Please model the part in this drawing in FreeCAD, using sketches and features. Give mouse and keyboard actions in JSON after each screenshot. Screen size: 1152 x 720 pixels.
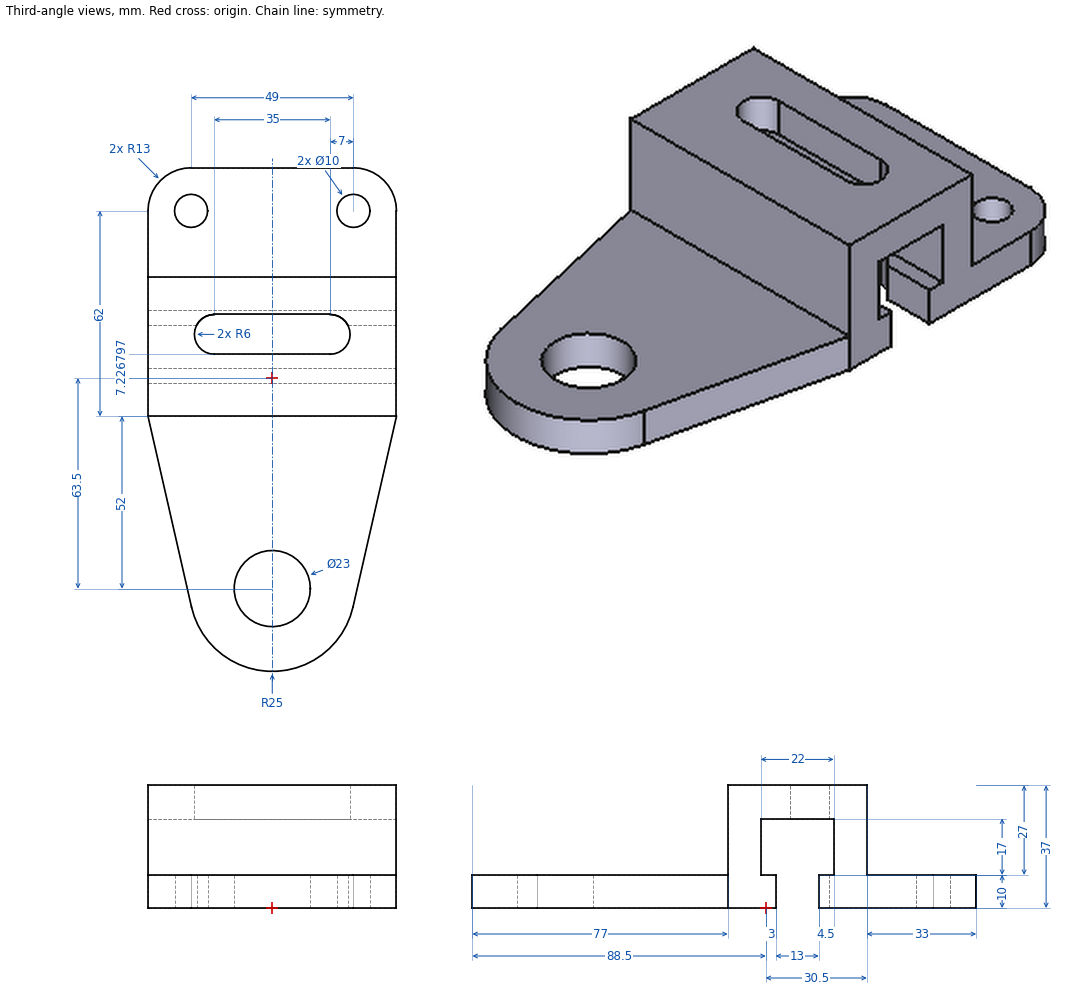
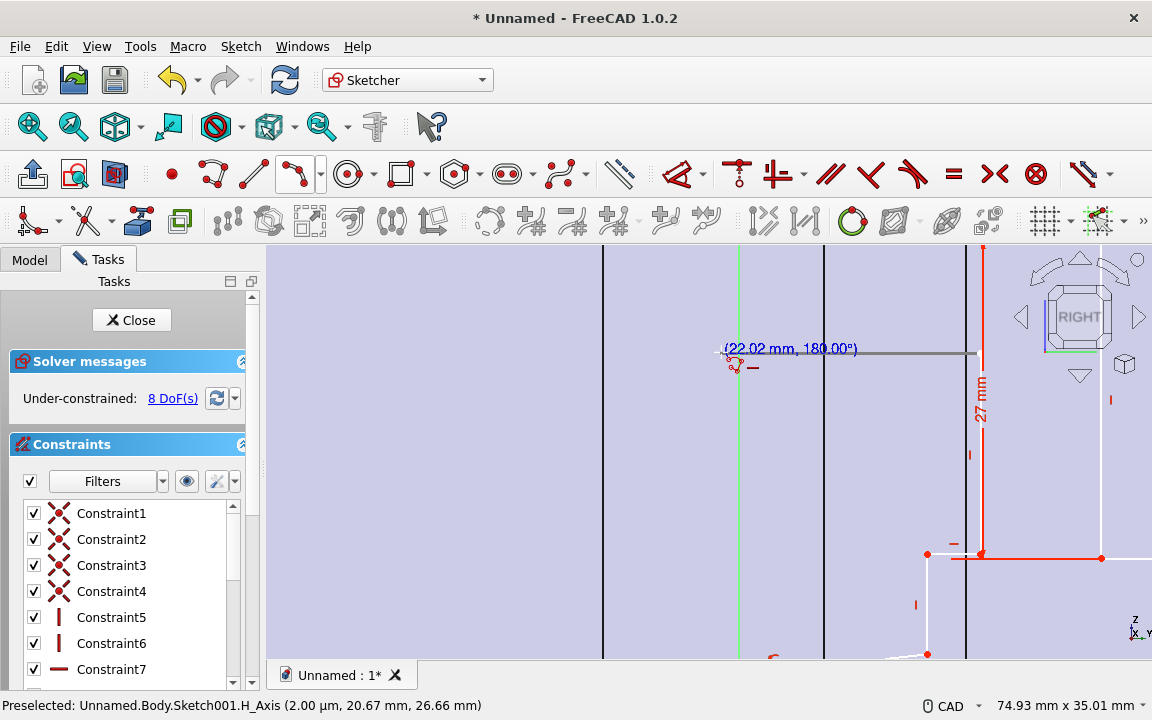
{"action": "left_click", "coordinate": [721, 352]}
{"action": "left_click", "coordinate": [721, 553]}
{"action": "left_click", "coordinate": [774, 553]}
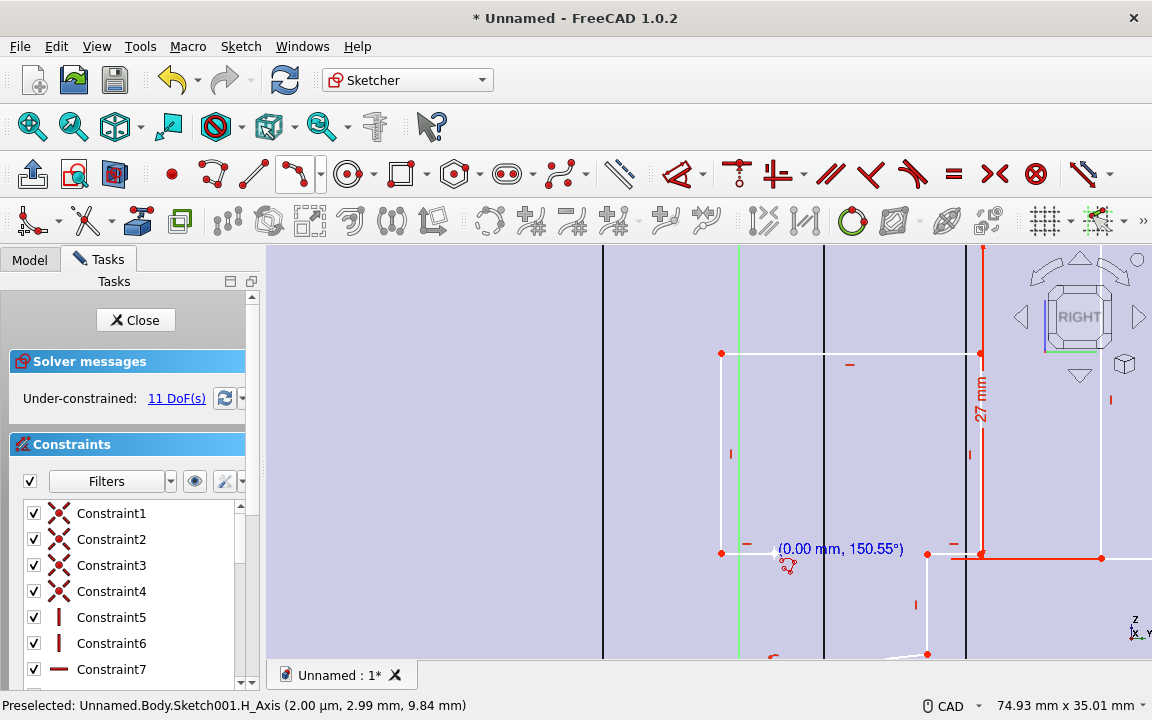
{"action": "scroll", "coordinate": [657, 452], "scroll_direction": "down", "scroll_amount": 7}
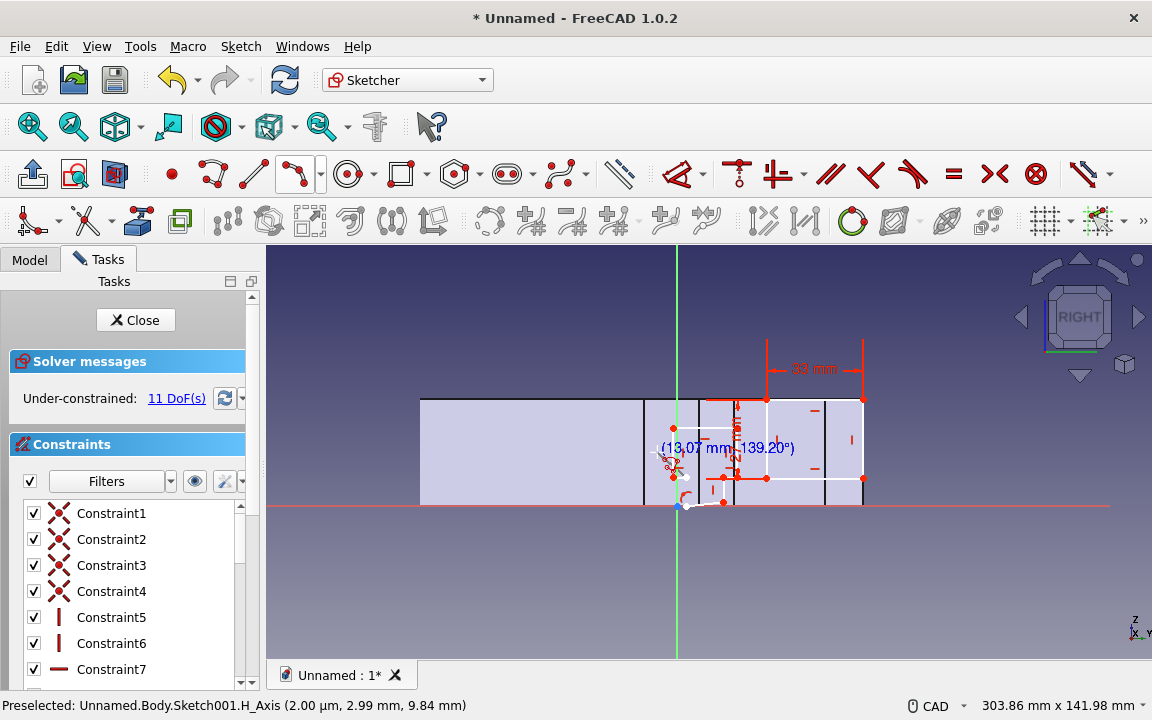
{"action": "scroll", "coordinate": [686, 506], "scroll_direction": "up", "scroll_amount": 3}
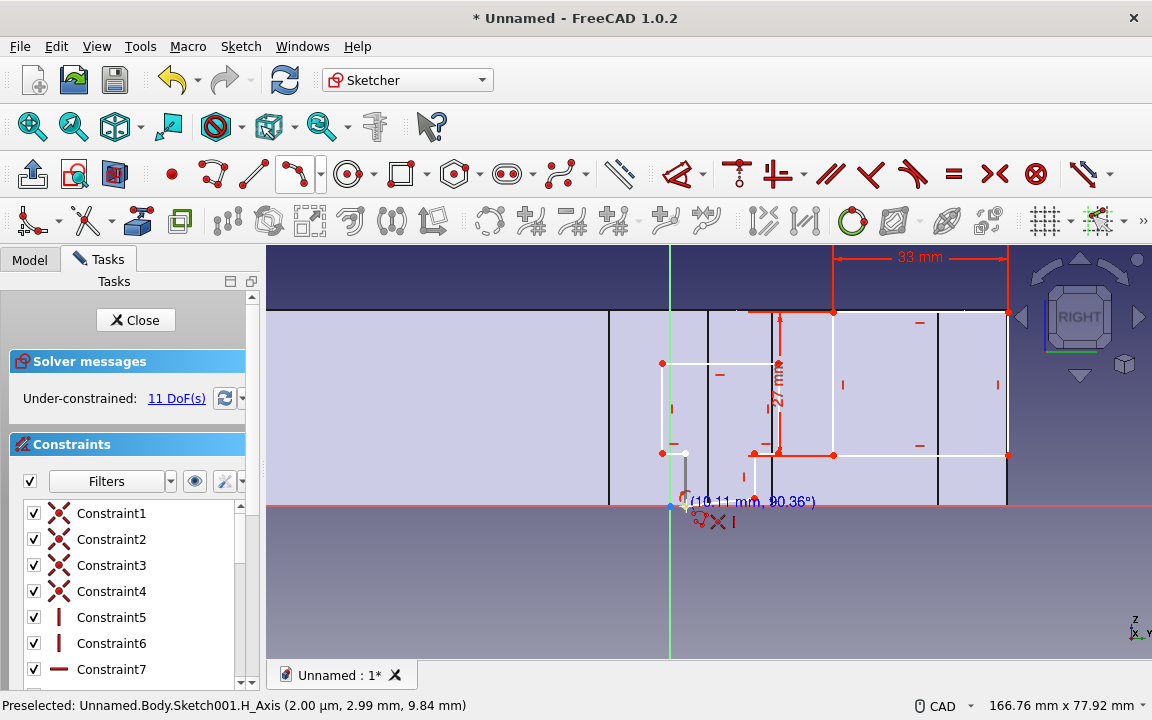
{"action": "left_click", "coordinate": [686, 506]}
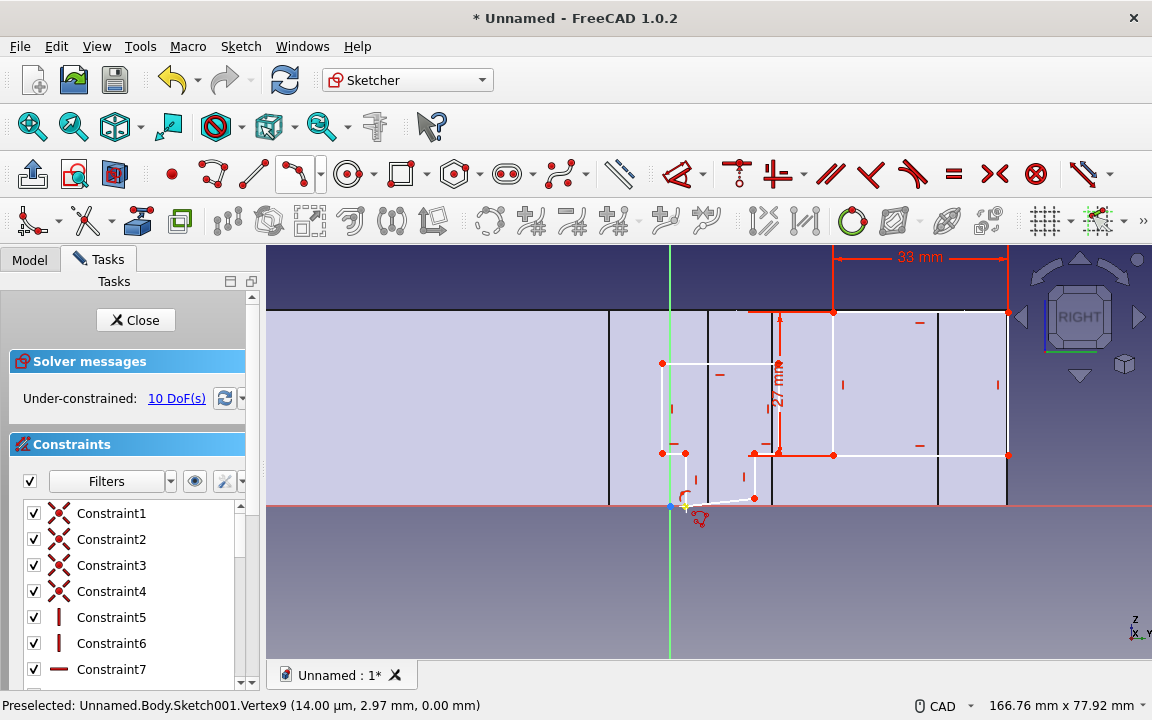
{"action": "left_click", "coordinate": [400, 174]}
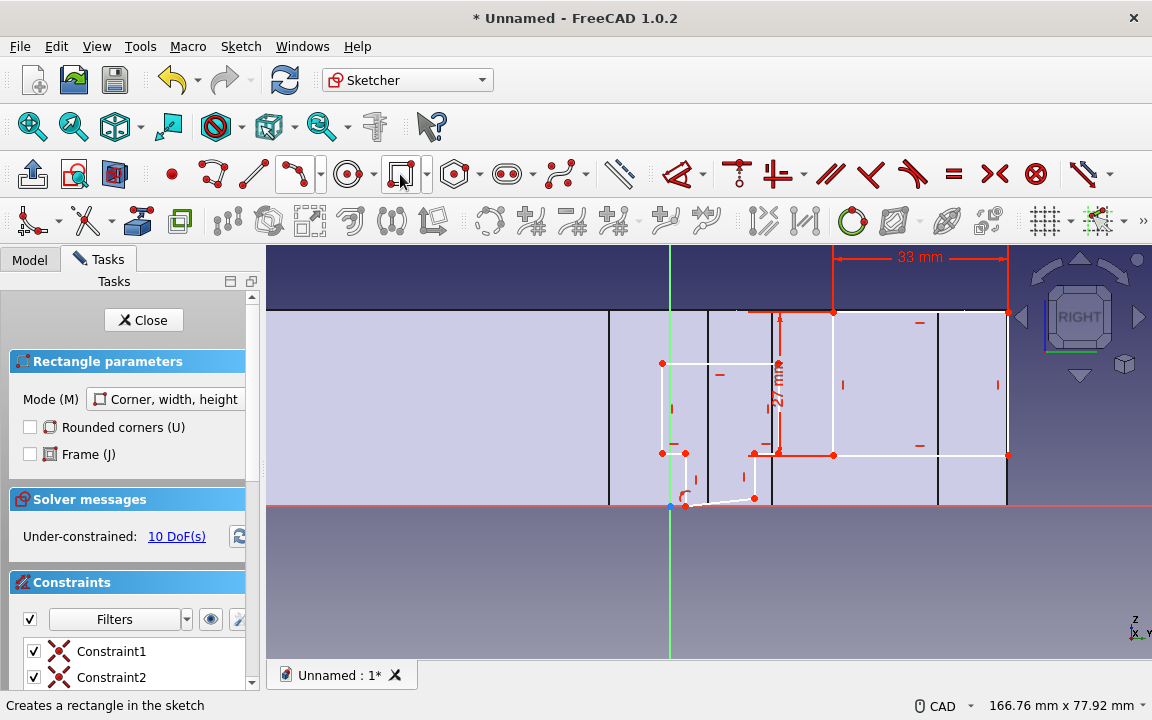
{"action": "scroll", "coordinate": [685, 505], "scroll_direction": "down", "scroll_amount": 3}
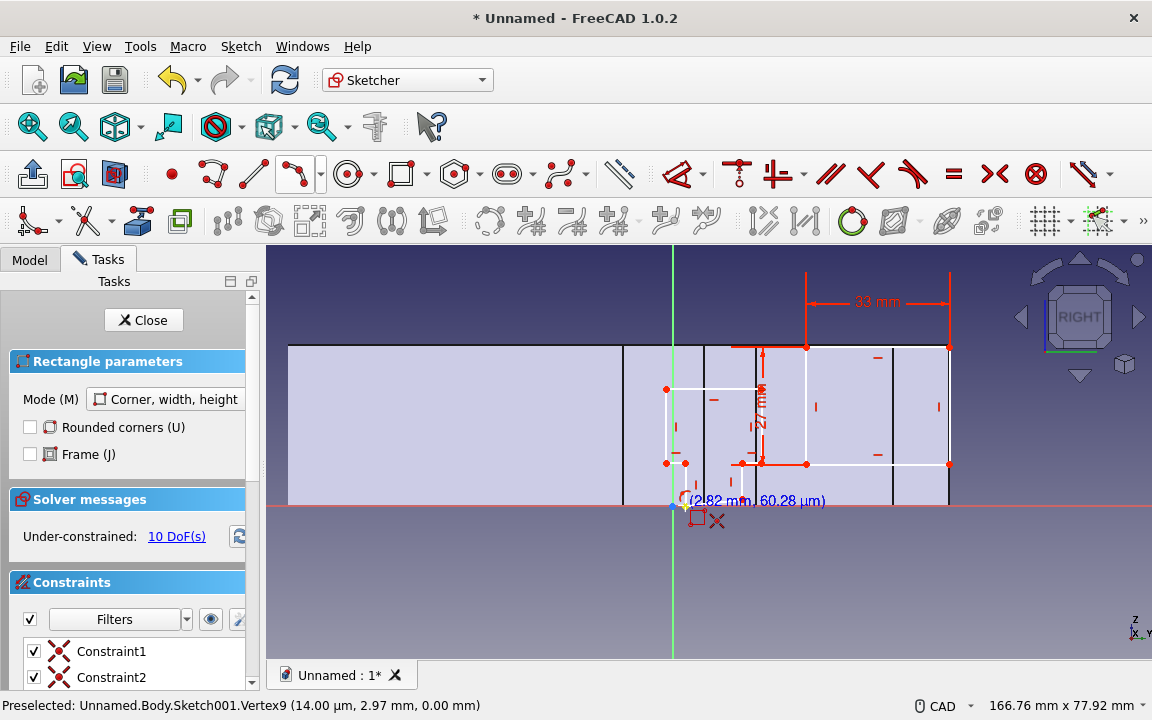
{"action": "left_click", "coordinate": [419, 398]}
{"action": "mouse_move", "coordinate": [643, 477]}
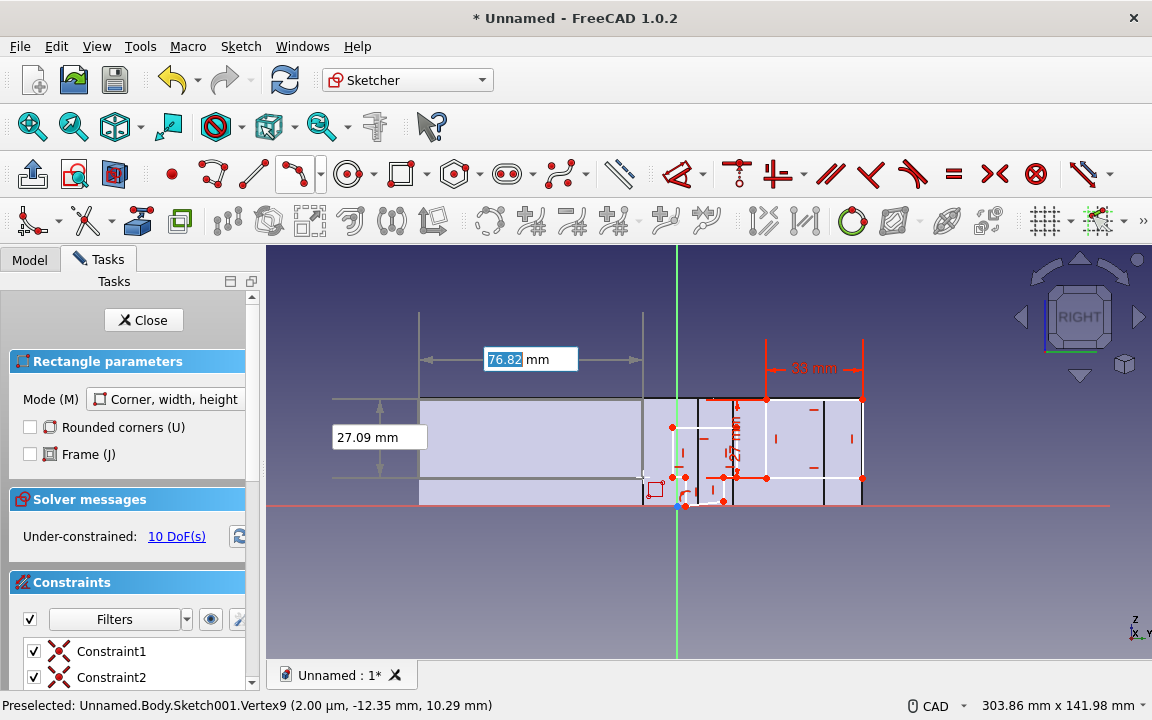
{"action": "type", "text": "77"}
{"action": "key", "text": "Tab"}
{"action": "type", "text": "27"}
{"action": "key", "text": "Return"}
{"action": "key", "text": "Escape"}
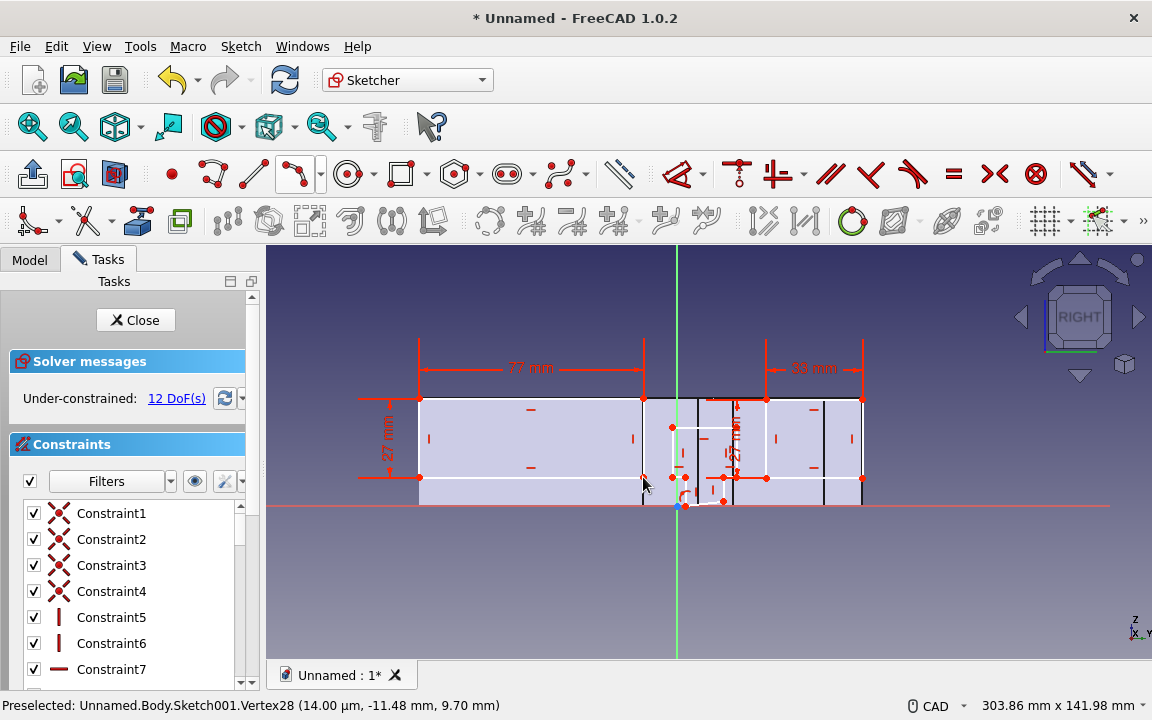
{"action": "left_click", "coordinate": [697, 505]}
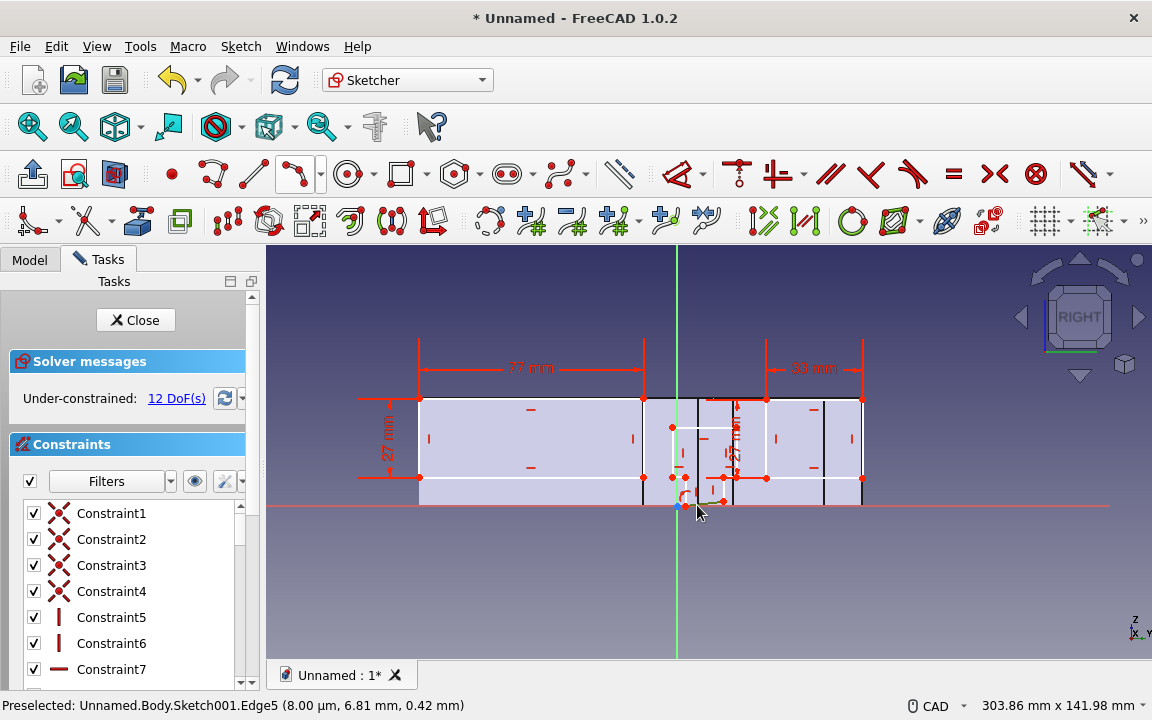
{"action": "left_click", "coordinate": [804, 174]}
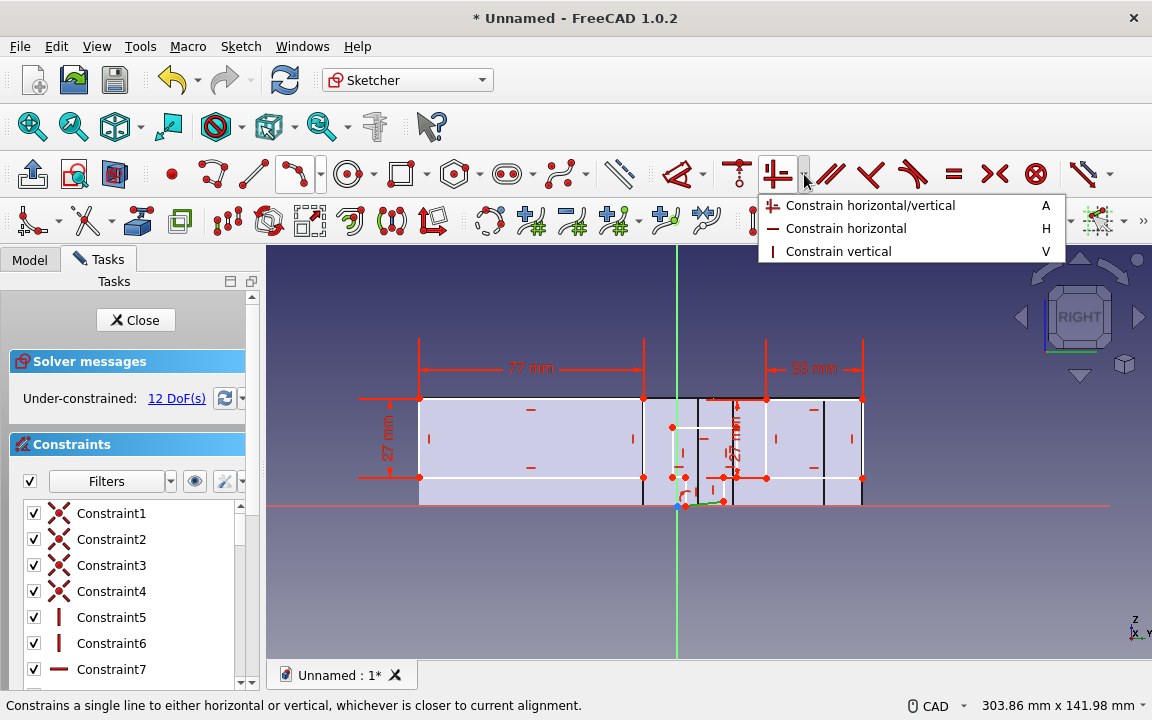
{"action": "left_click", "coordinate": [912, 228]}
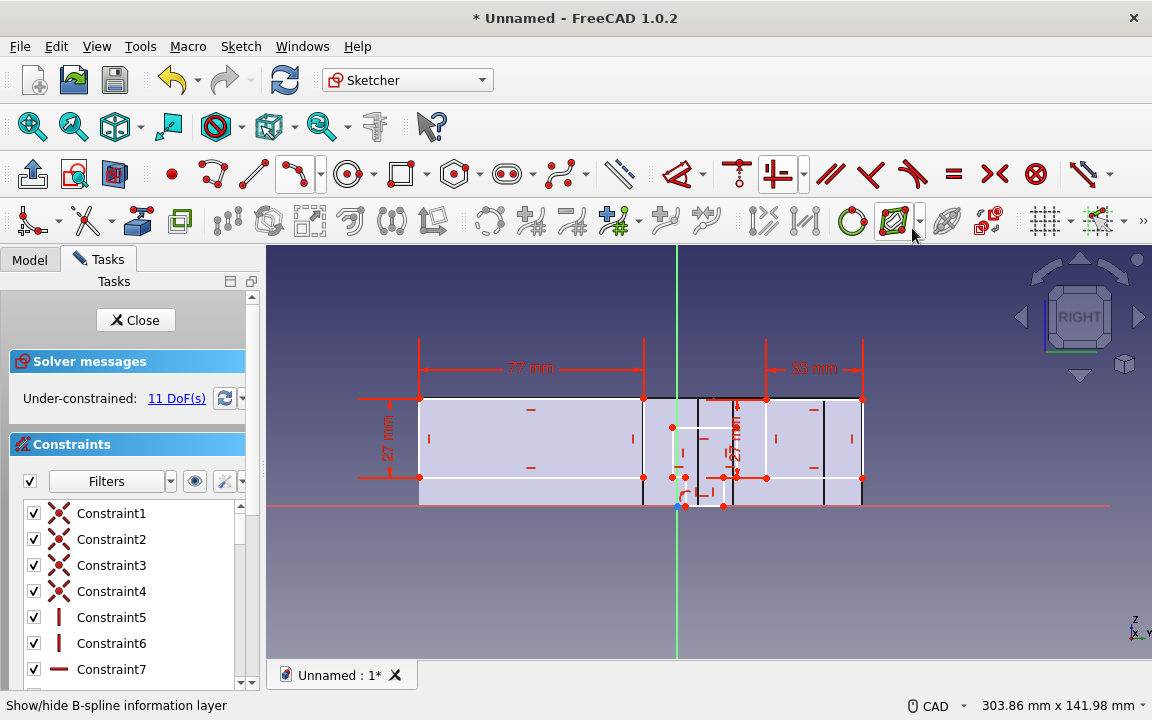
{"action": "left_click", "coordinate": [676, 174]}